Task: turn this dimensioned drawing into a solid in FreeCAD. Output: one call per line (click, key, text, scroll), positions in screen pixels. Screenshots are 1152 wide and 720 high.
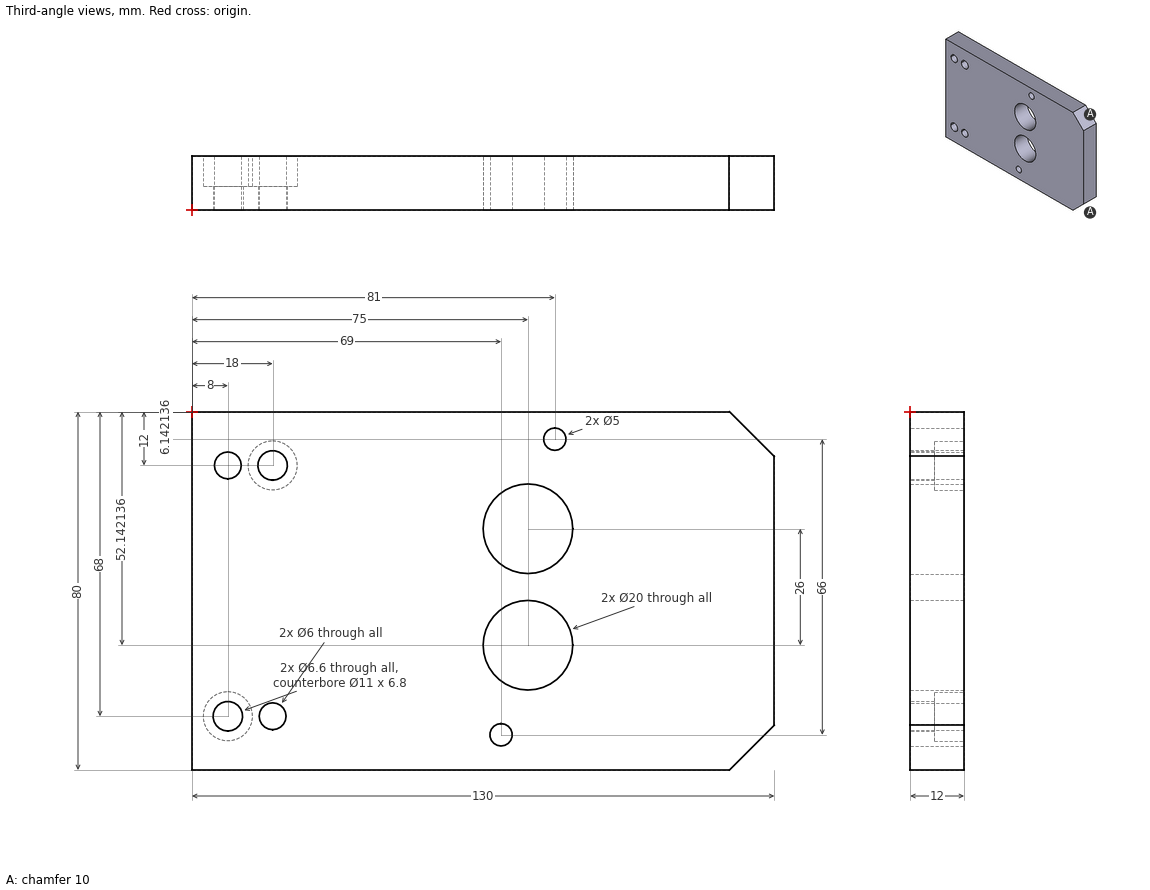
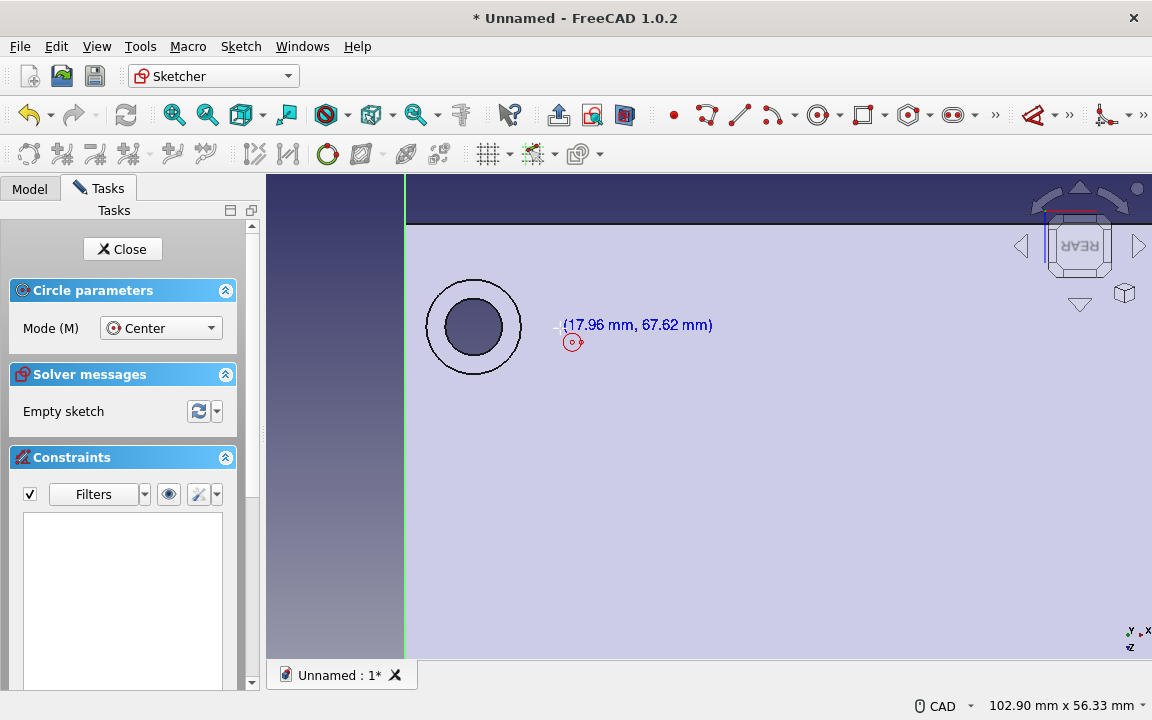
click(560, 327)
click(578, 309)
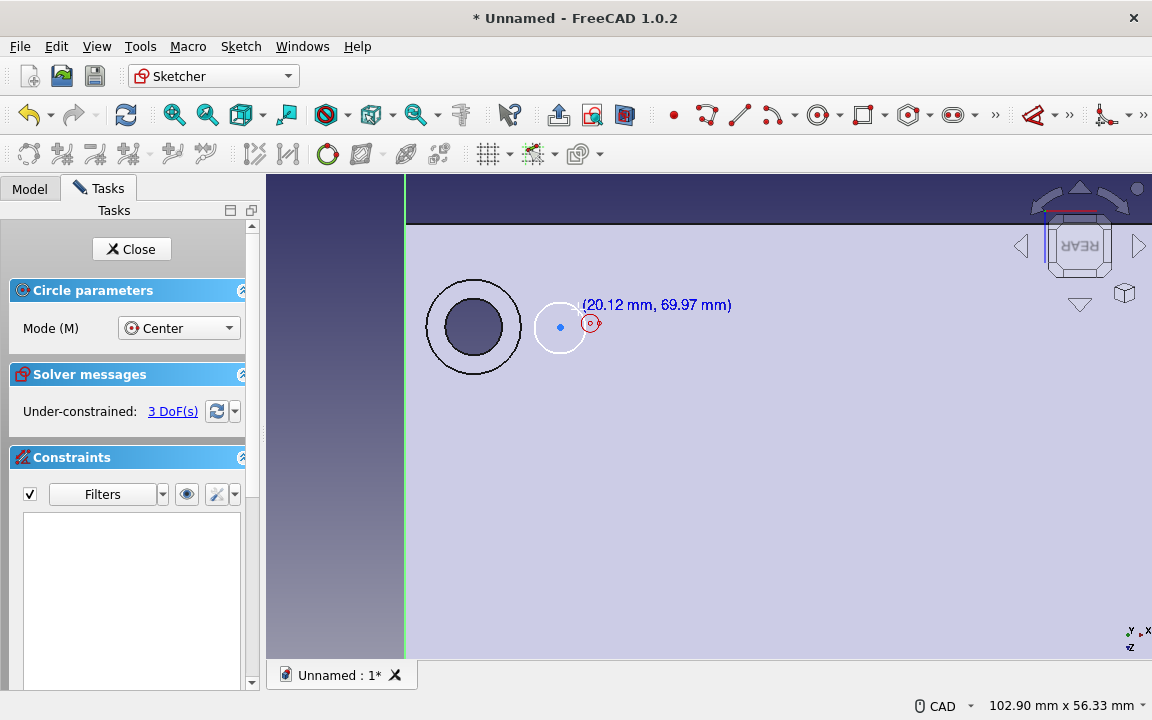
scroll(759, 261, down, 4)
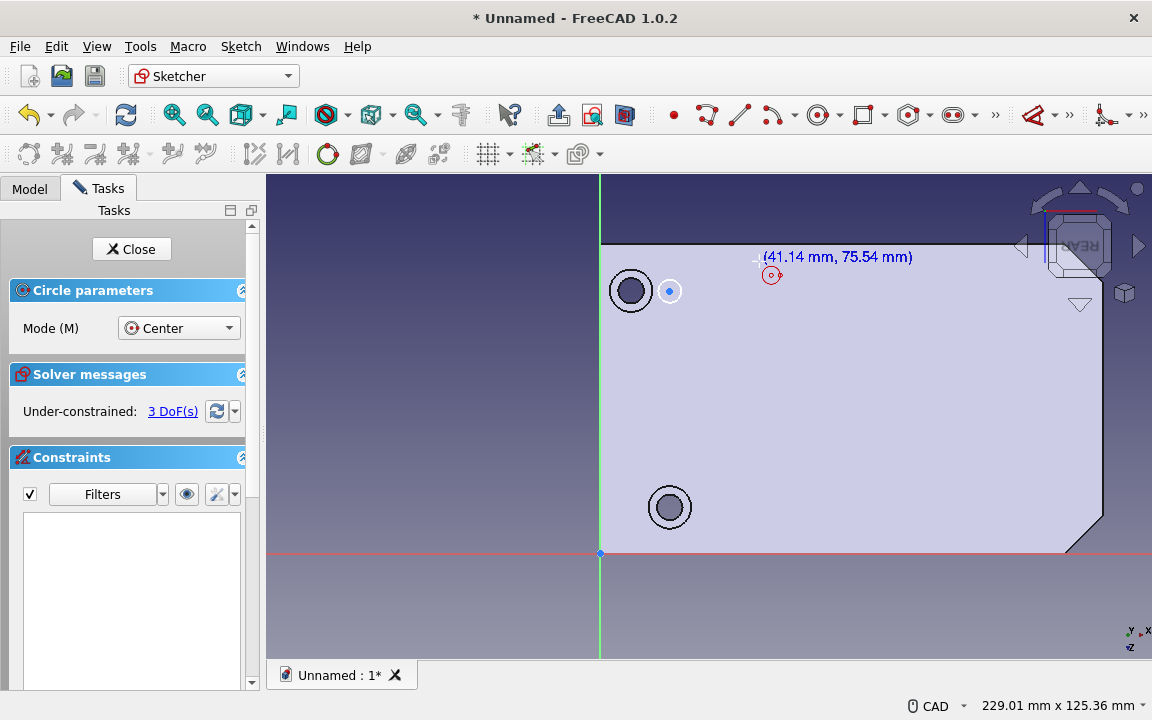
scroll(631, 507, up, 4)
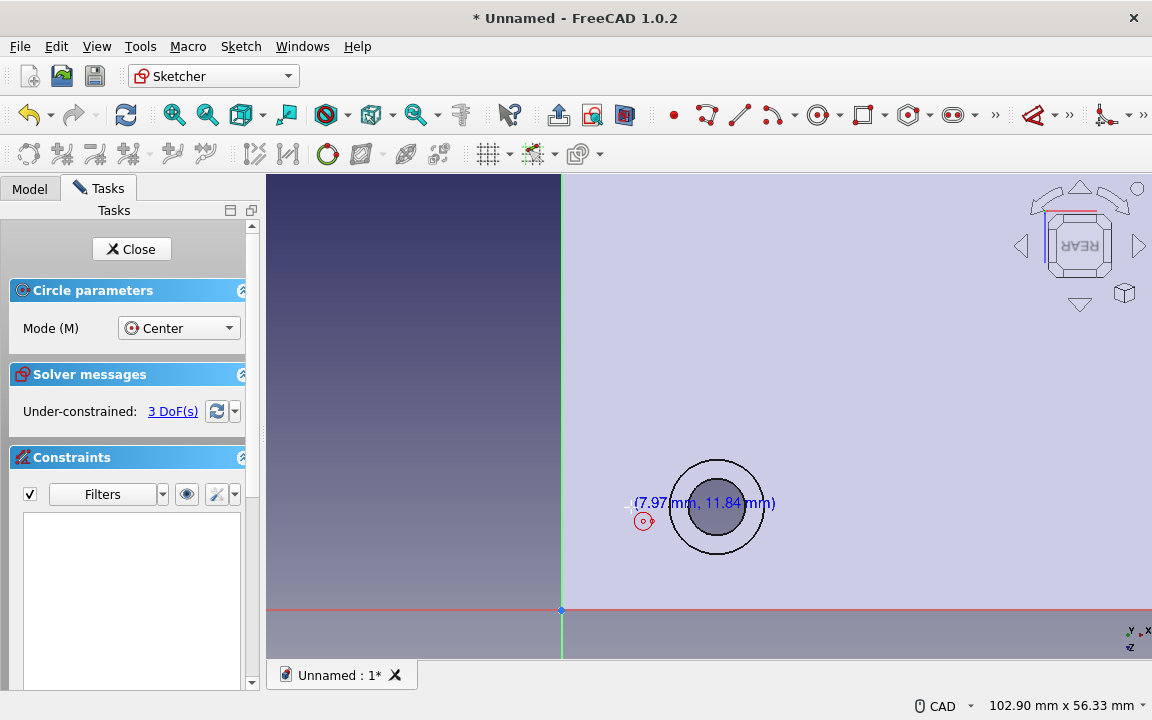
click(631, 507)
click(649, 489)
key(Escape)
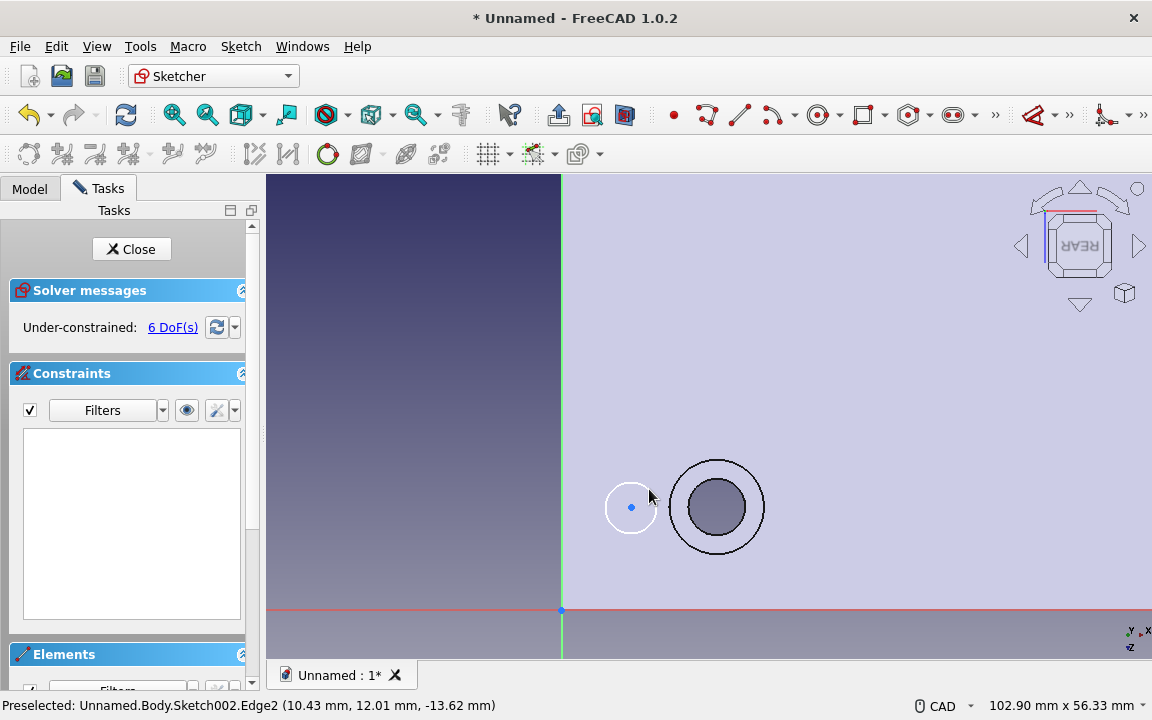
scroll(631, 508, down, 4)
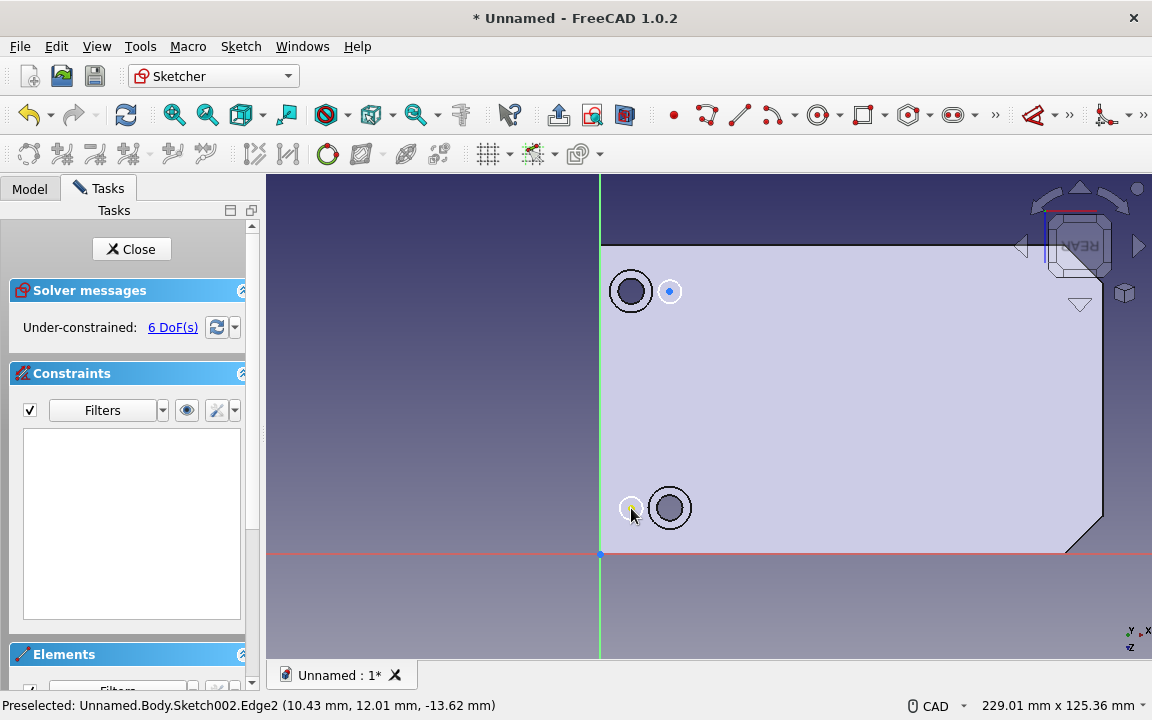
click(678, 284)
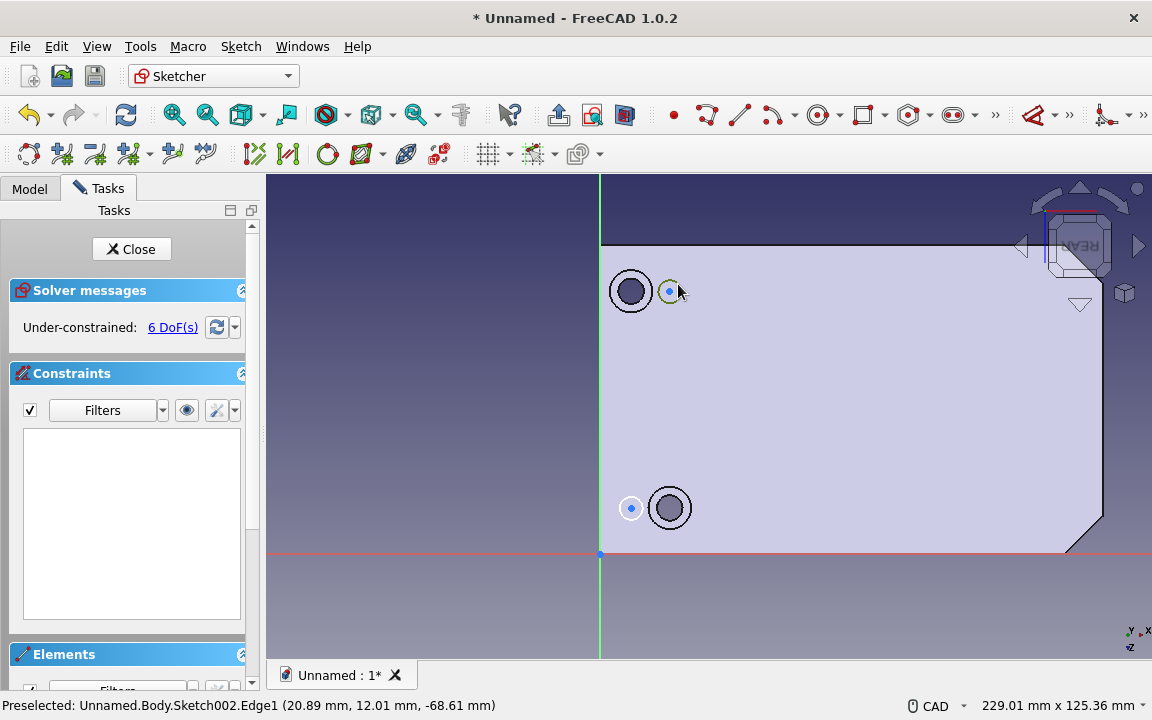
click(639, 500)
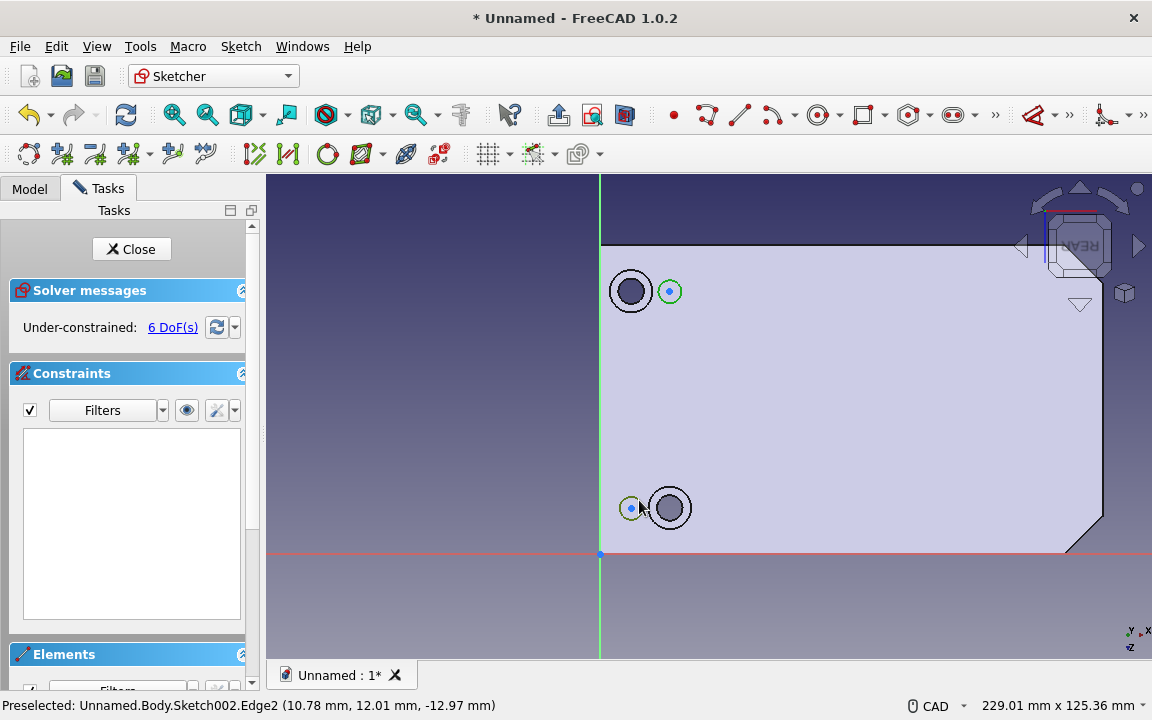
key(e)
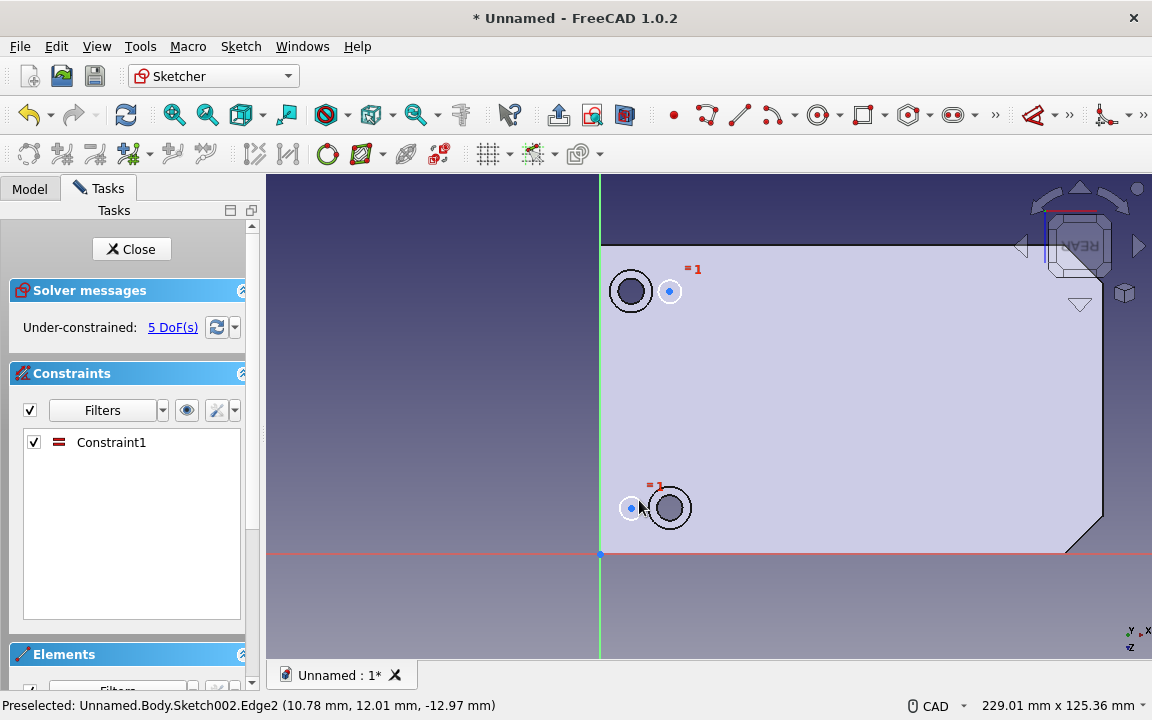
key(d)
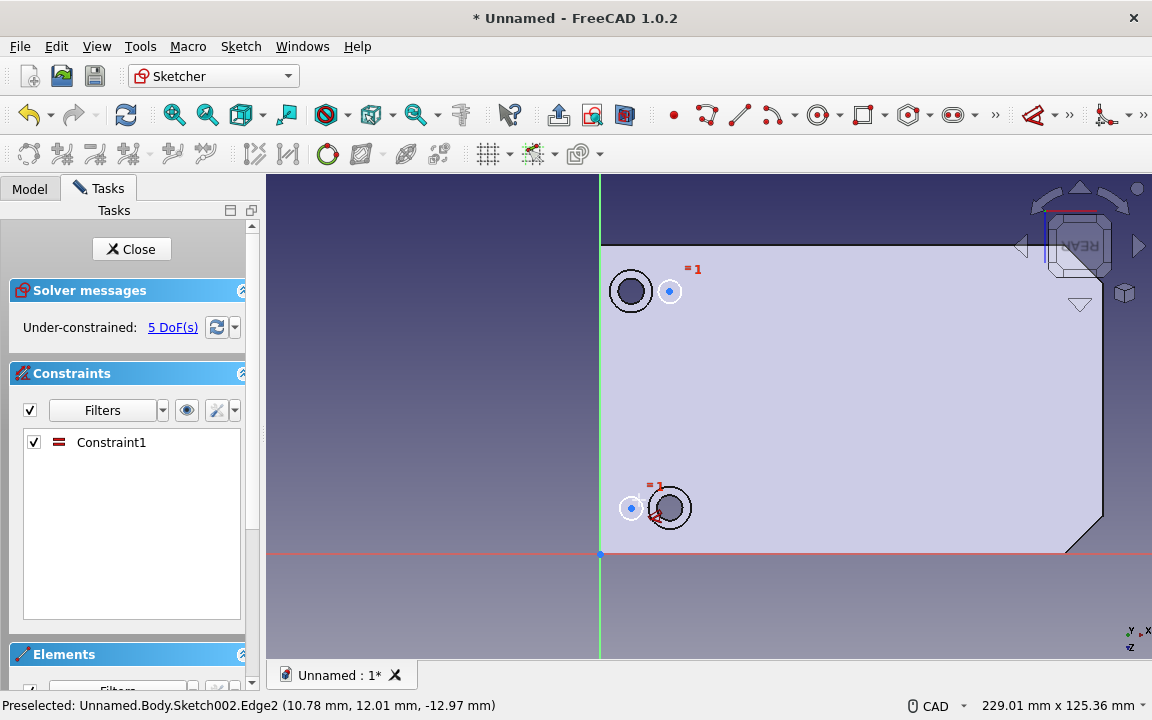
scroll(678, 284, up, 3)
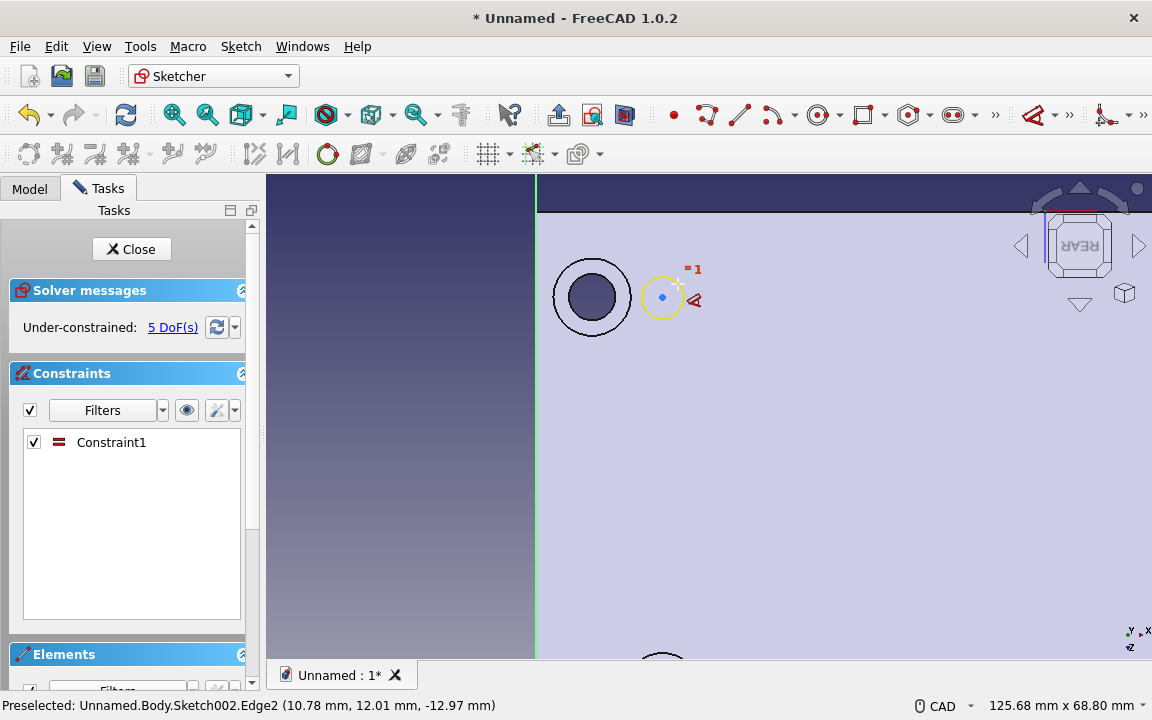
click(678, 283)
click(701, 261)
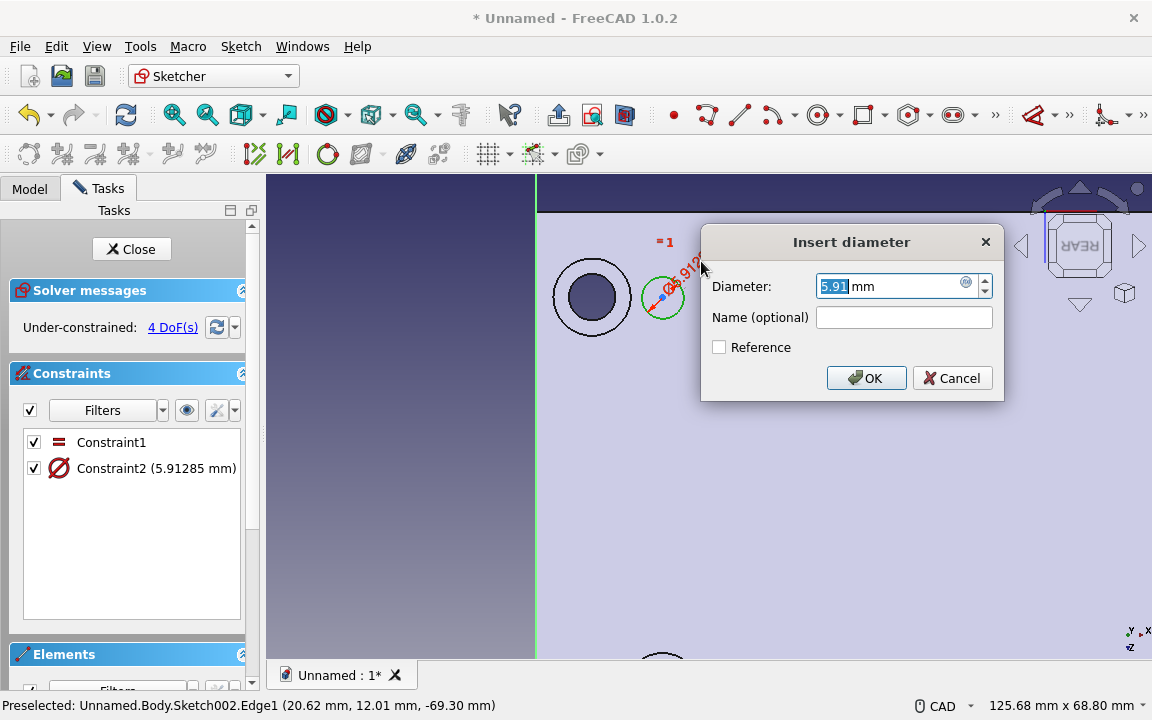
text(6)
key(Return)